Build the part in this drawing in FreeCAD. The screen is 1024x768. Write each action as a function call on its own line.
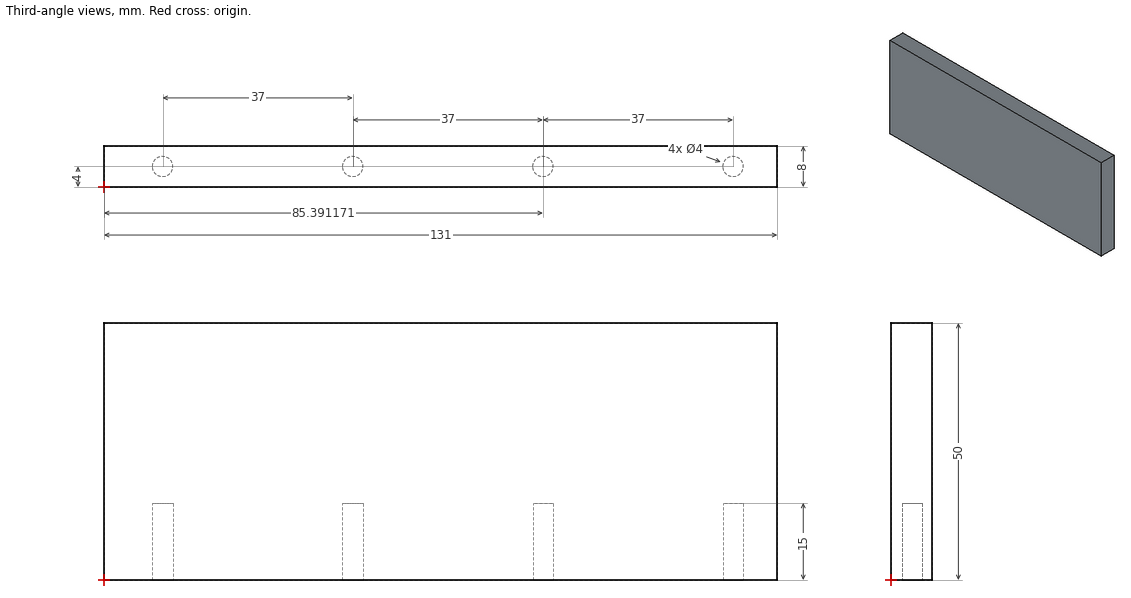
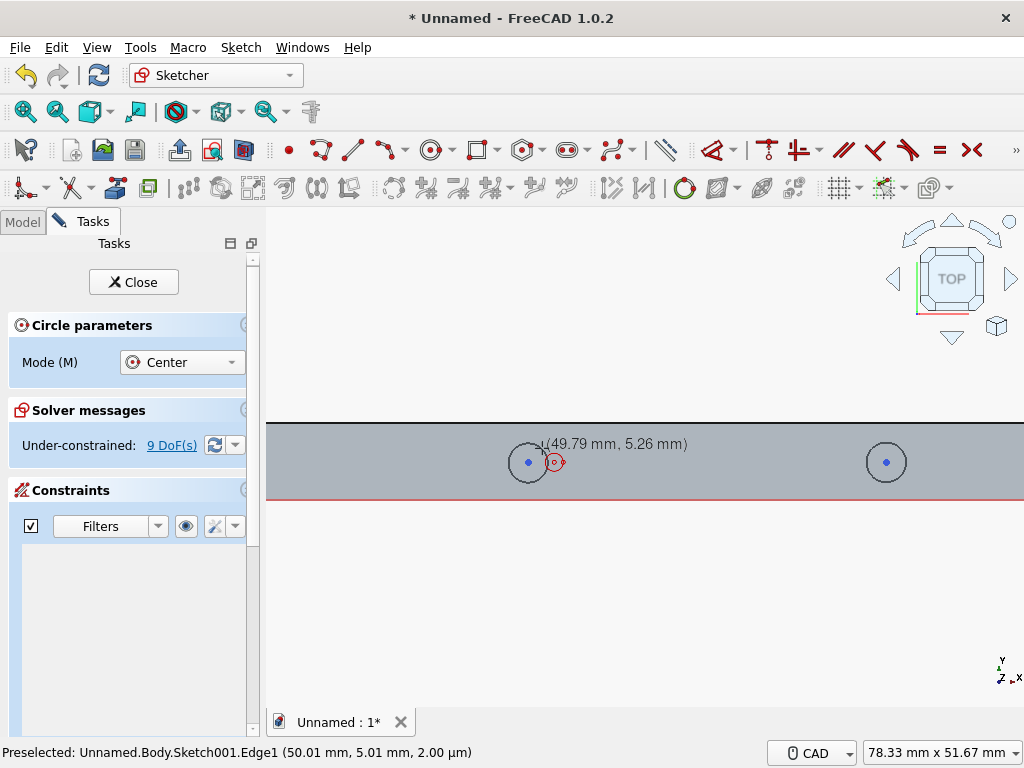
scroll(540, 451, down, 6)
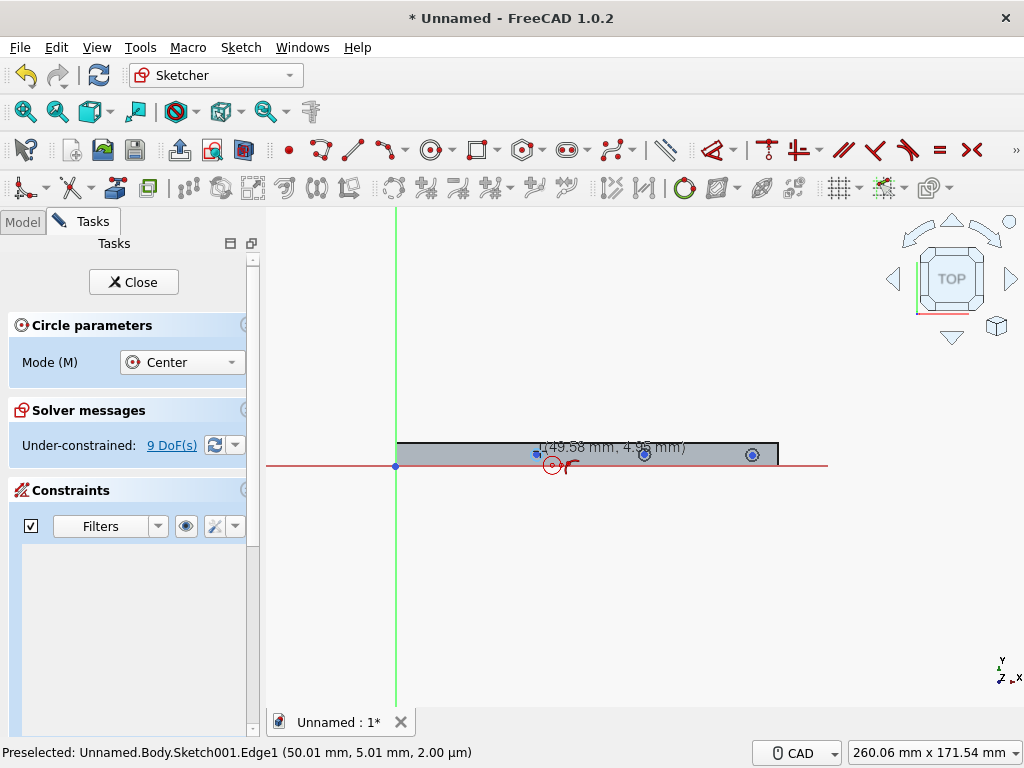
scroll(429, 454, up, 7)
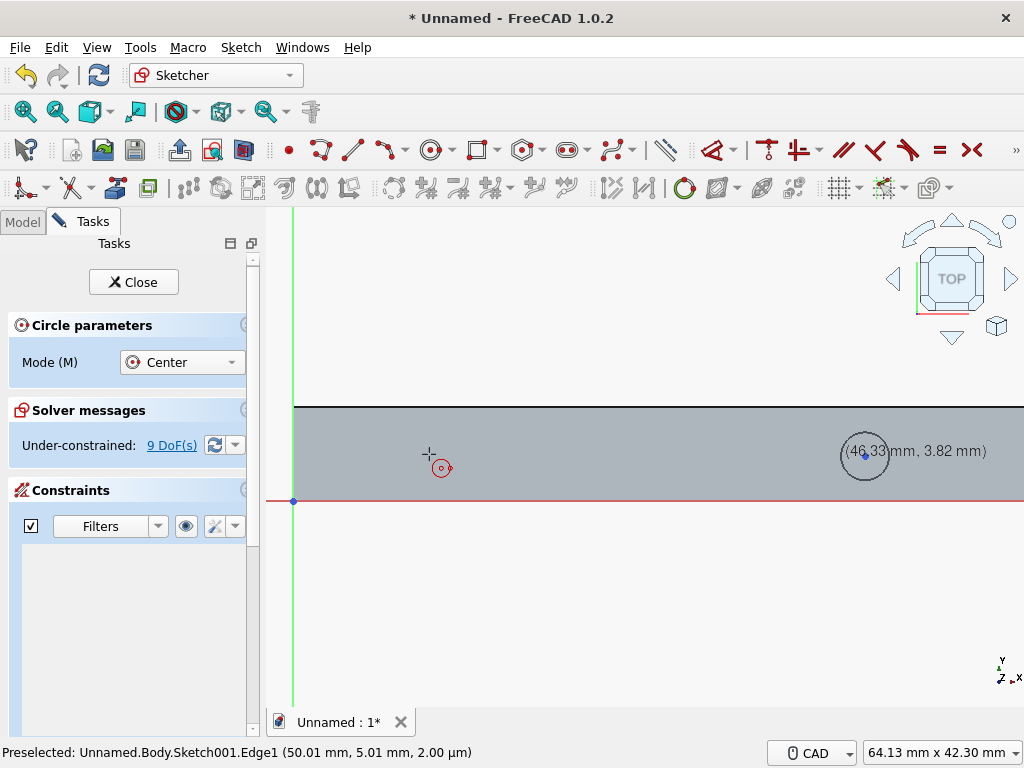
scroll(429, 454, down, 7)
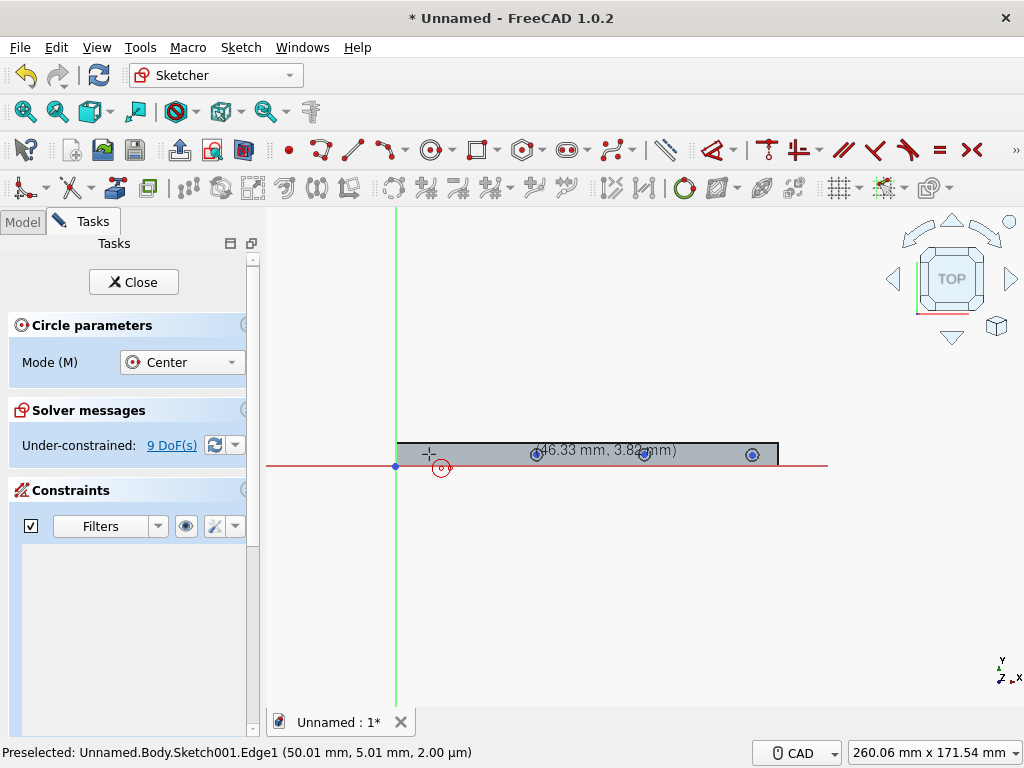
scroll(429, 454, up, 2)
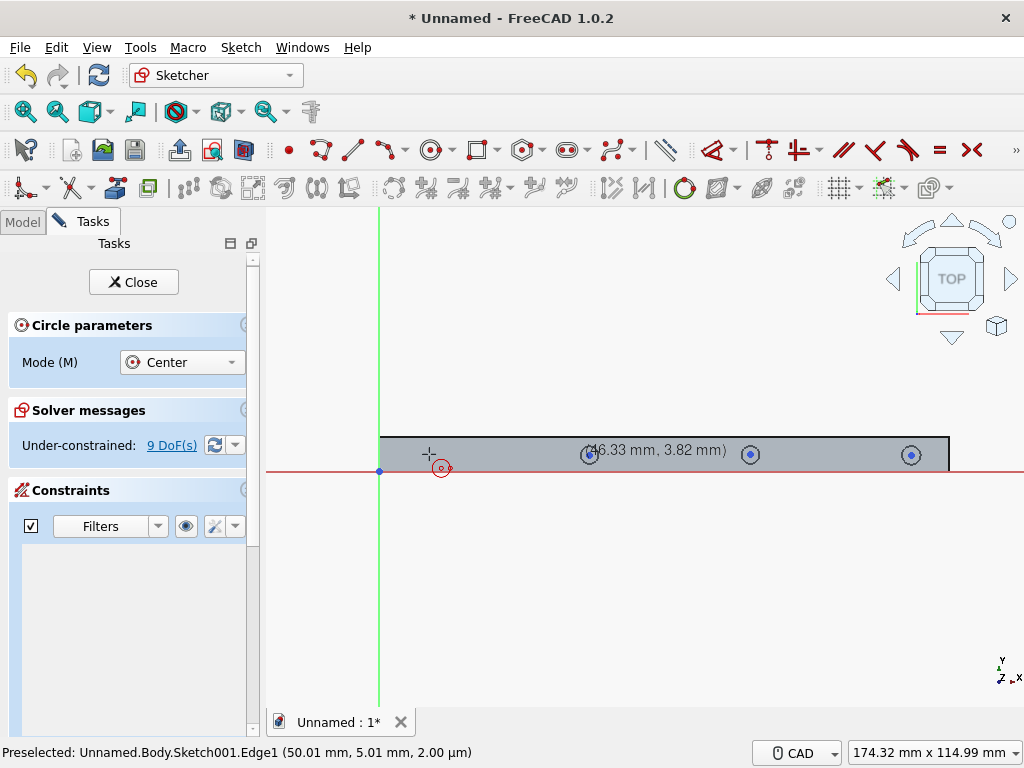
click(429, 454)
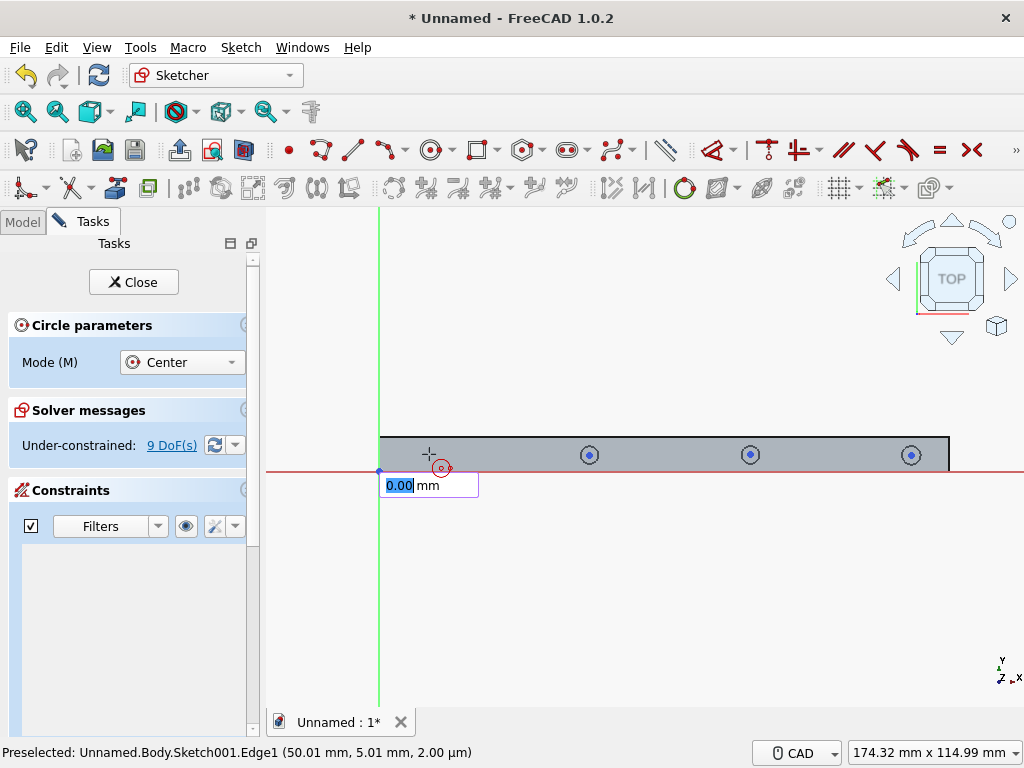
scroll(435, 448, up, 4)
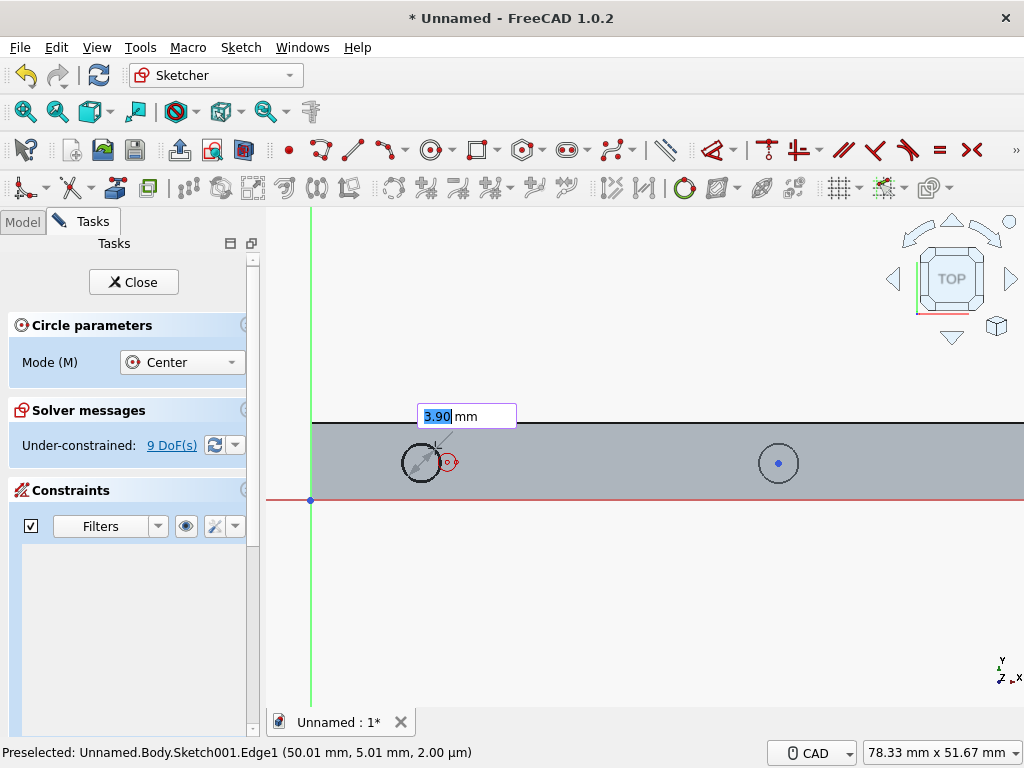
click(435, 448)
key(Escape)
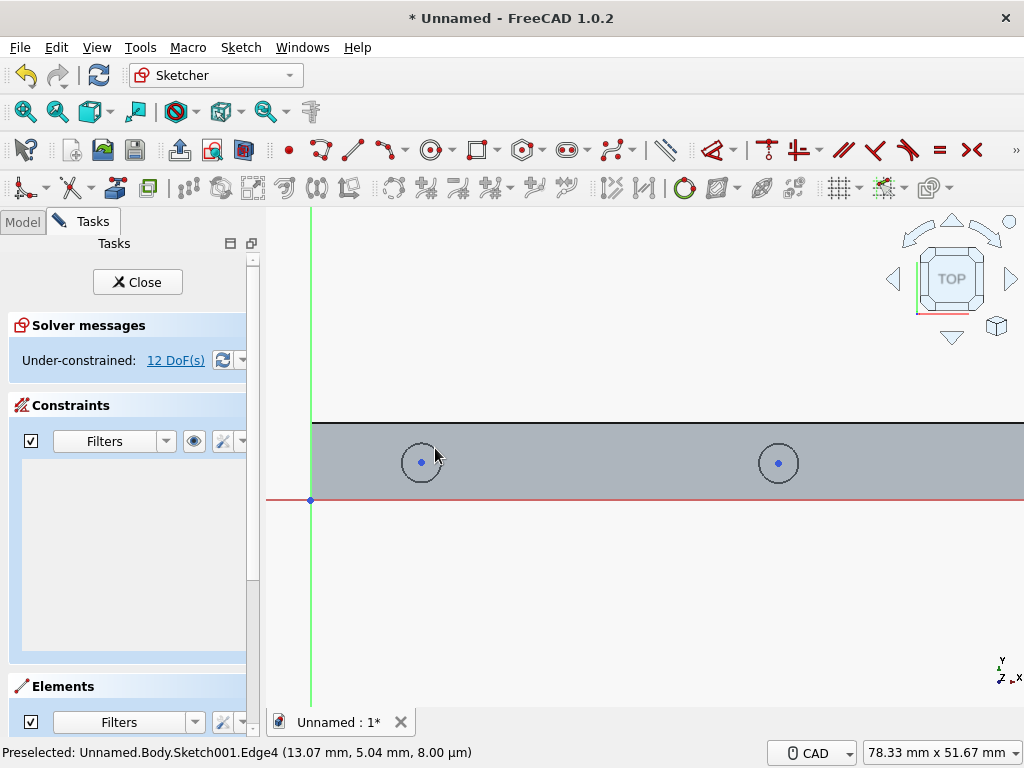
scroll(432, 451, down, 6)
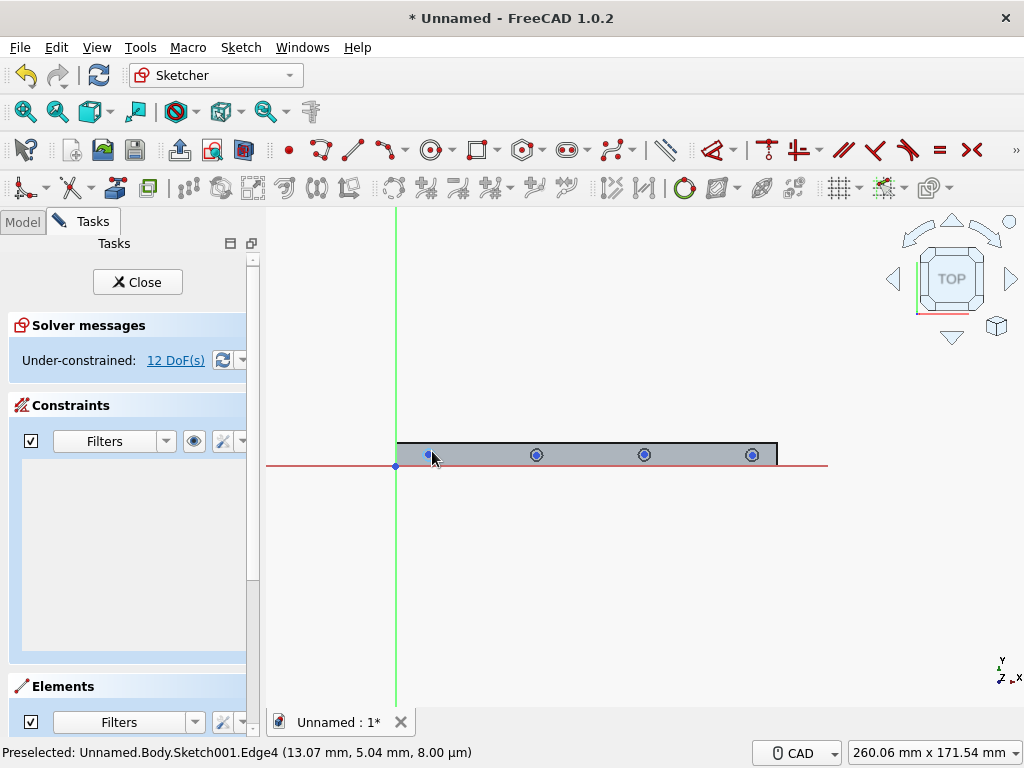
scroll(757, 451, up, 4)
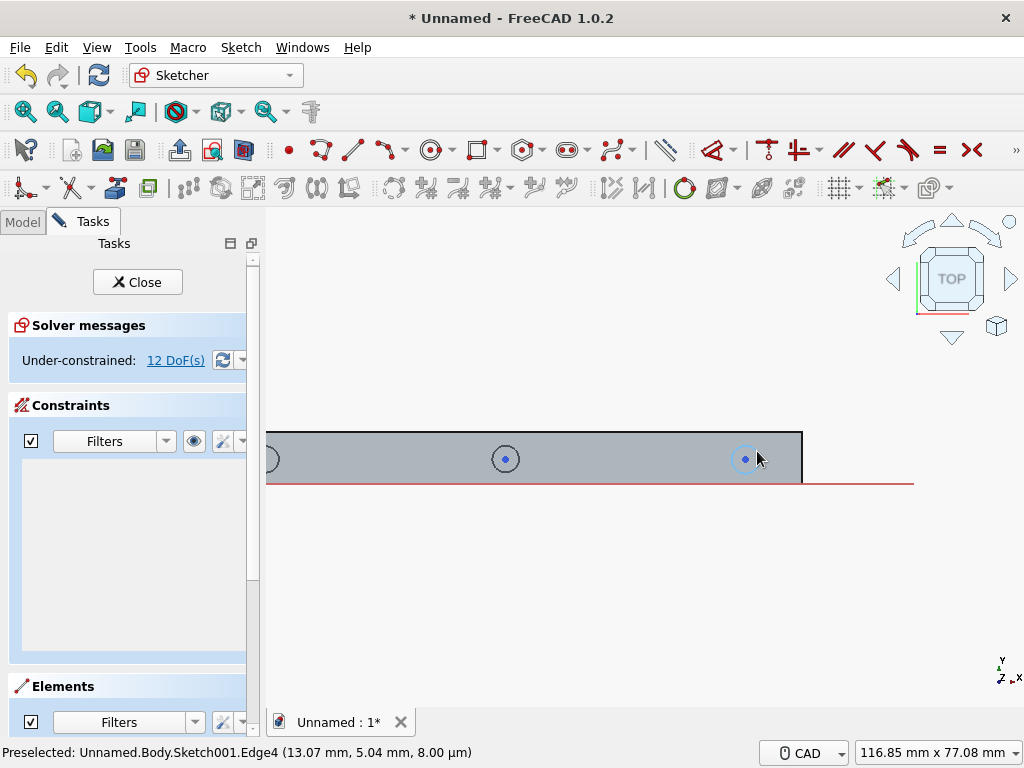
click(755, 450)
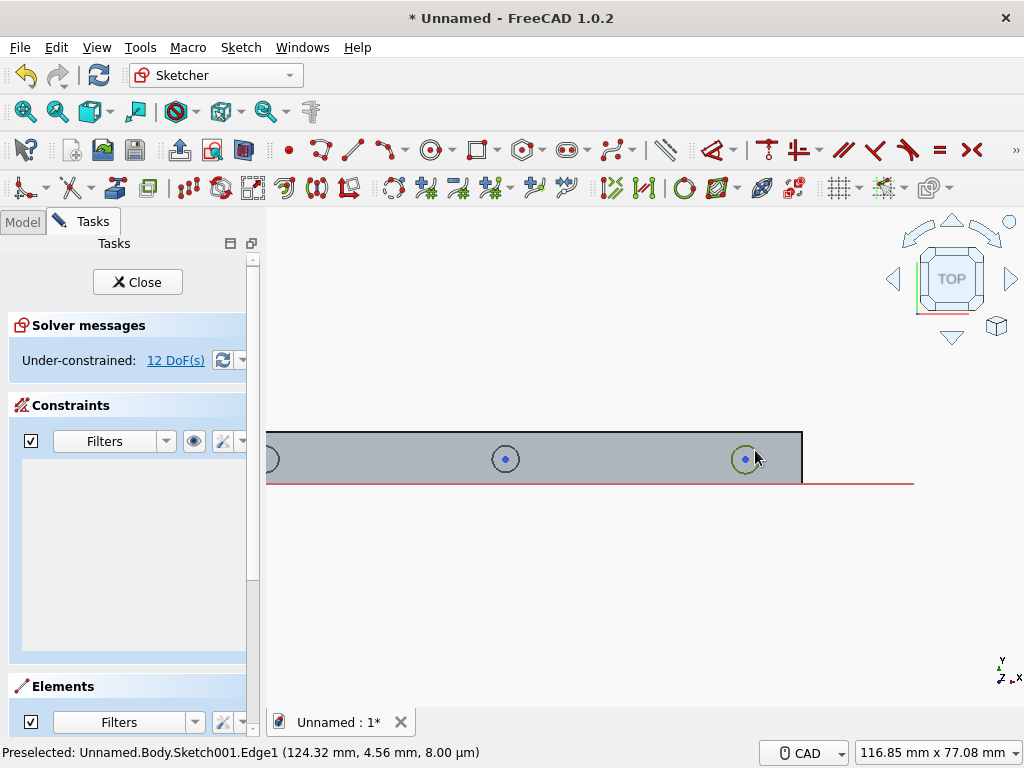
click(515, 450)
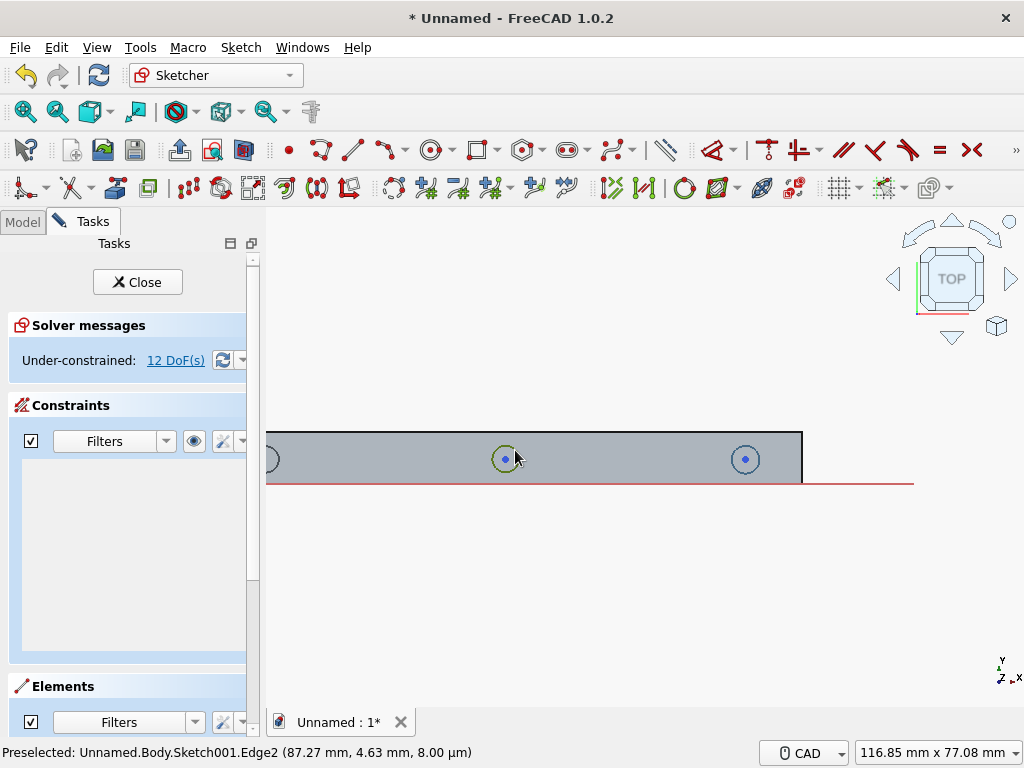
scroll(757, 451, down, 4)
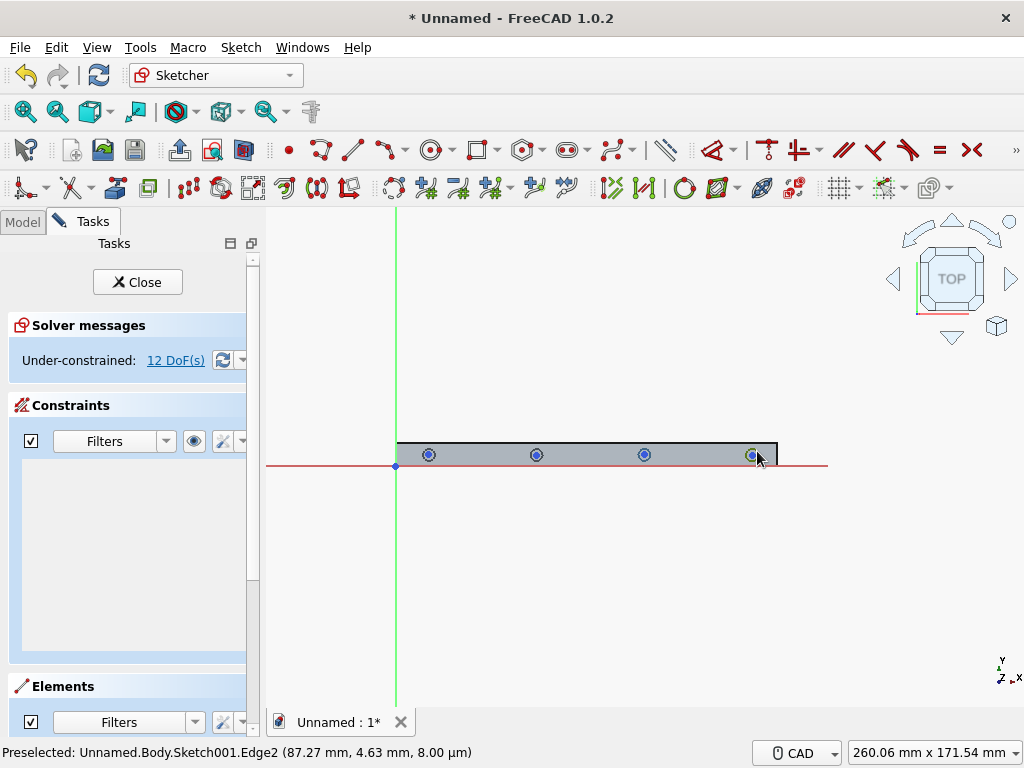
scroll(541, 451, up, 5)